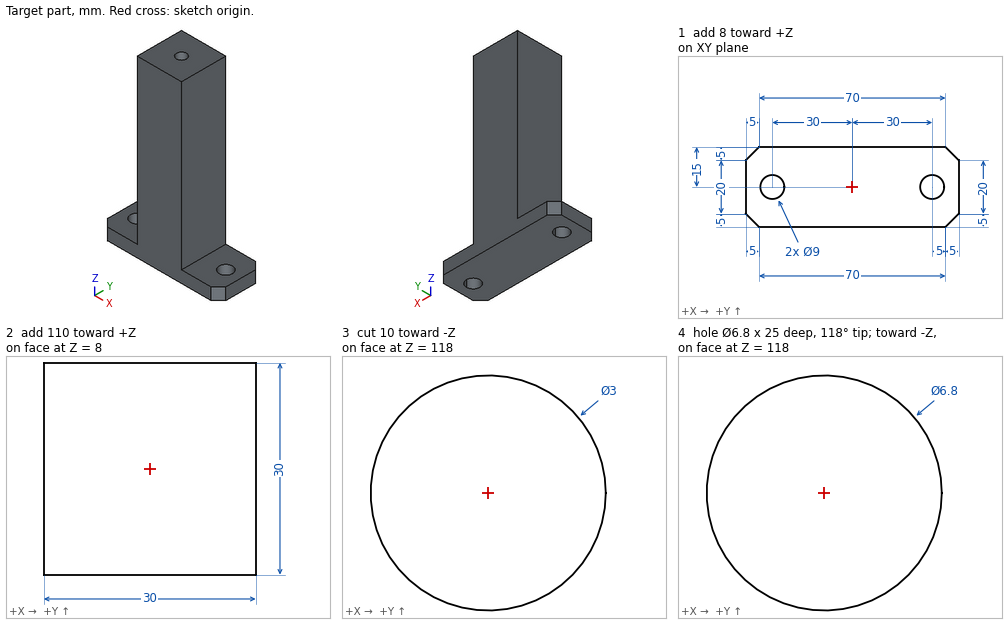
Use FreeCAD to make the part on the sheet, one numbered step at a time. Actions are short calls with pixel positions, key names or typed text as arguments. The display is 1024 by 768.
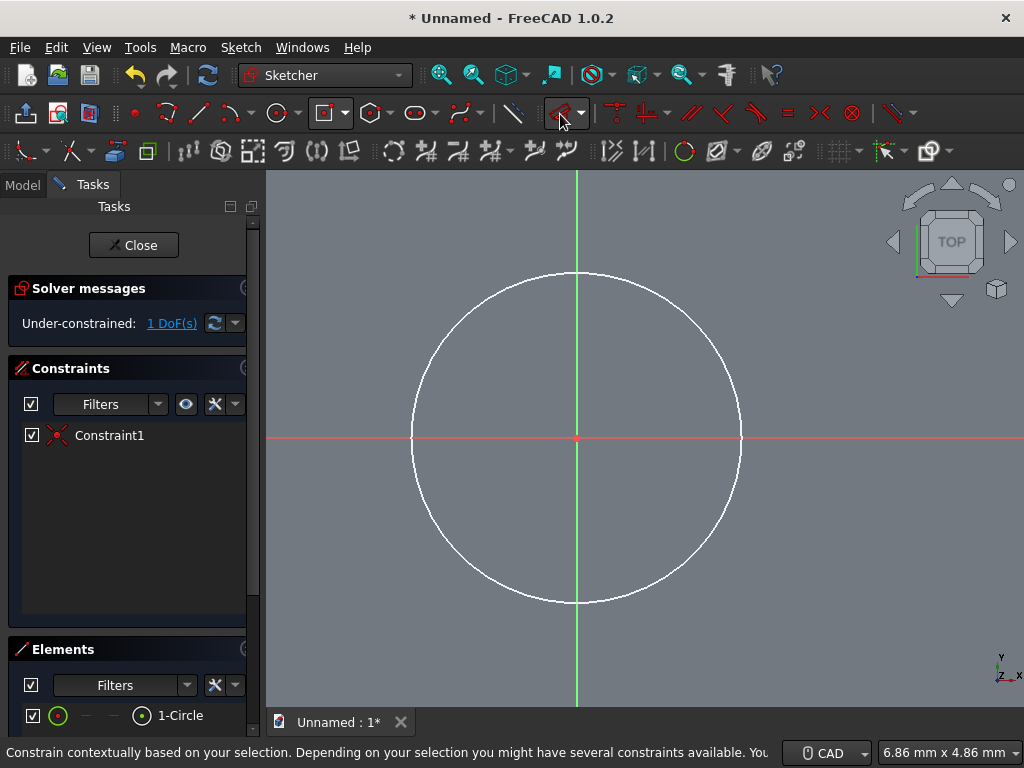
click(693, 321)
click(716, 298)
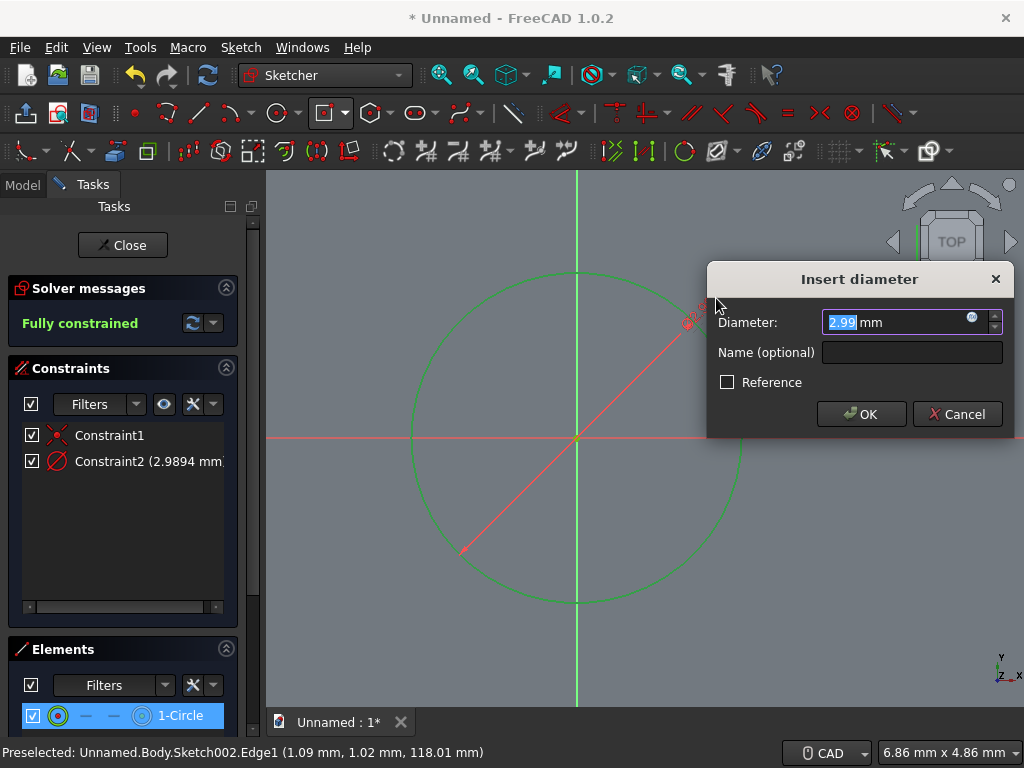
text(3)
key(Return)
key(Escape)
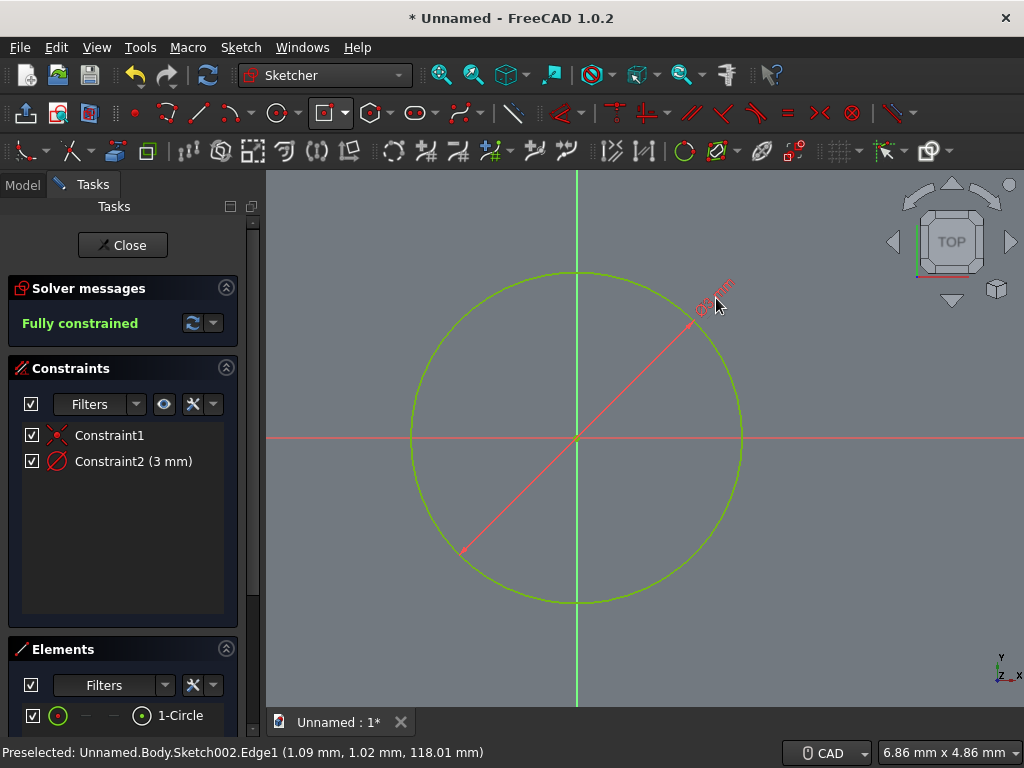
click(123, 245)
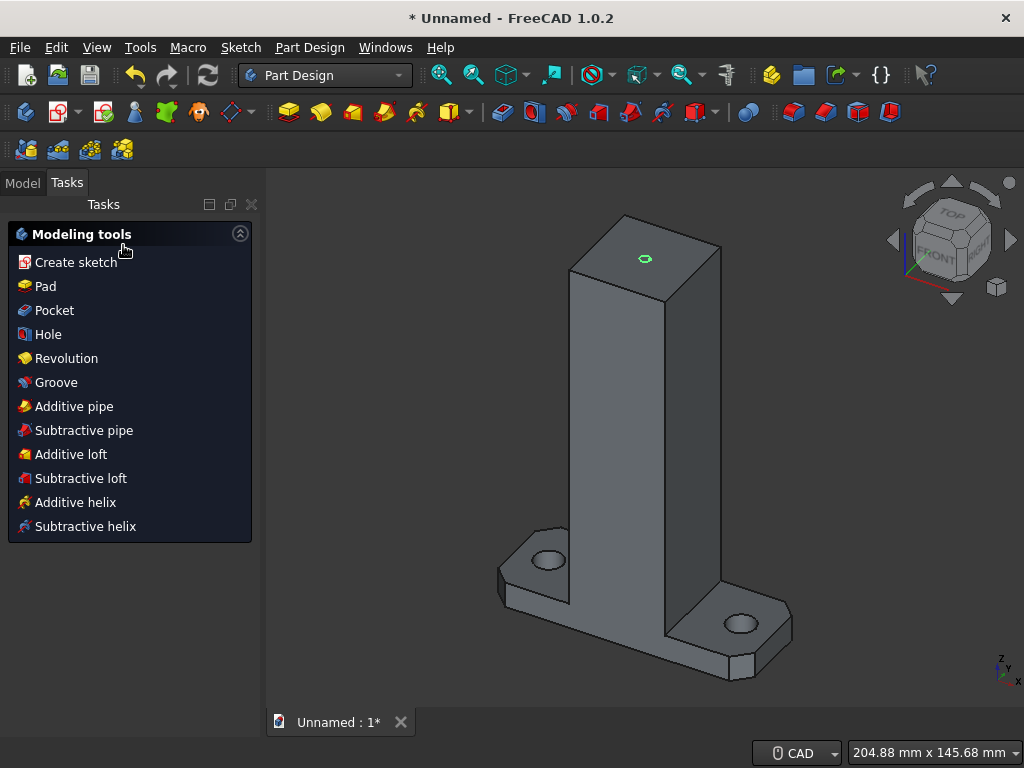
click(504, 112)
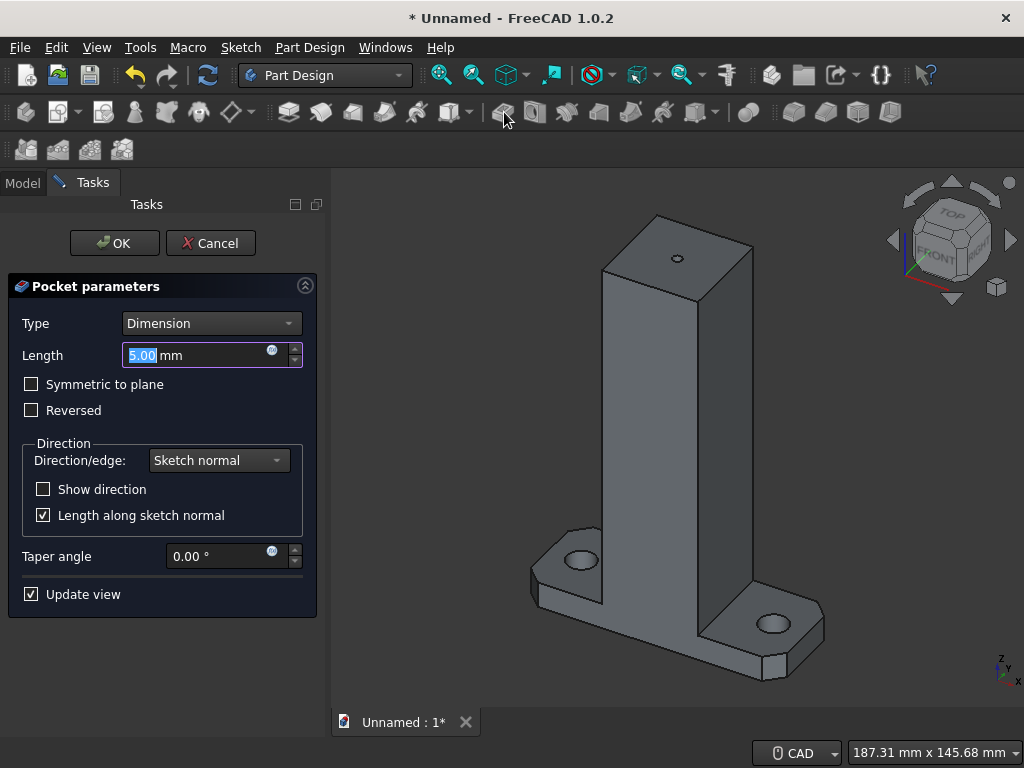
text(10)
key(Tab)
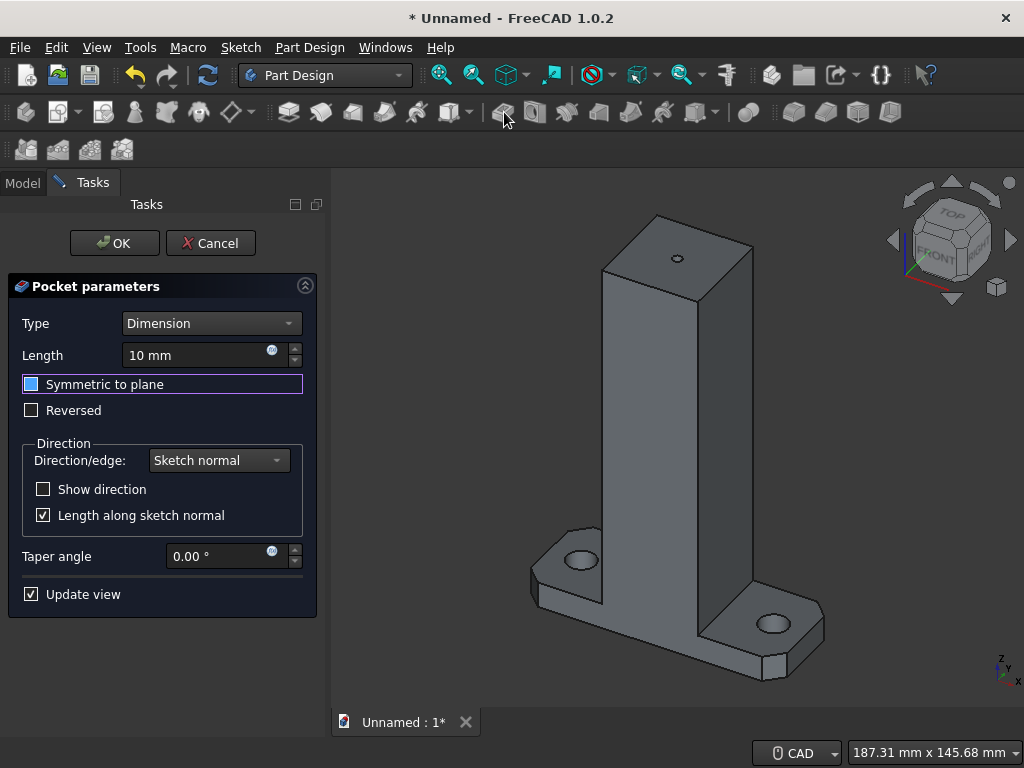
click(115, 243)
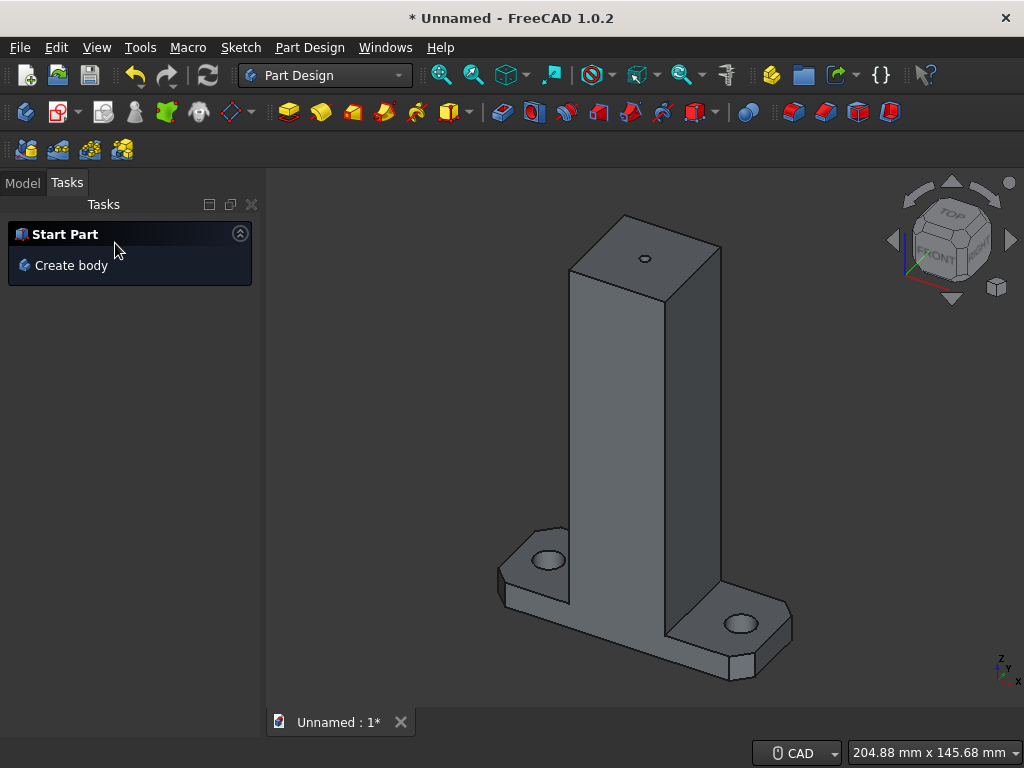
click(643, 278)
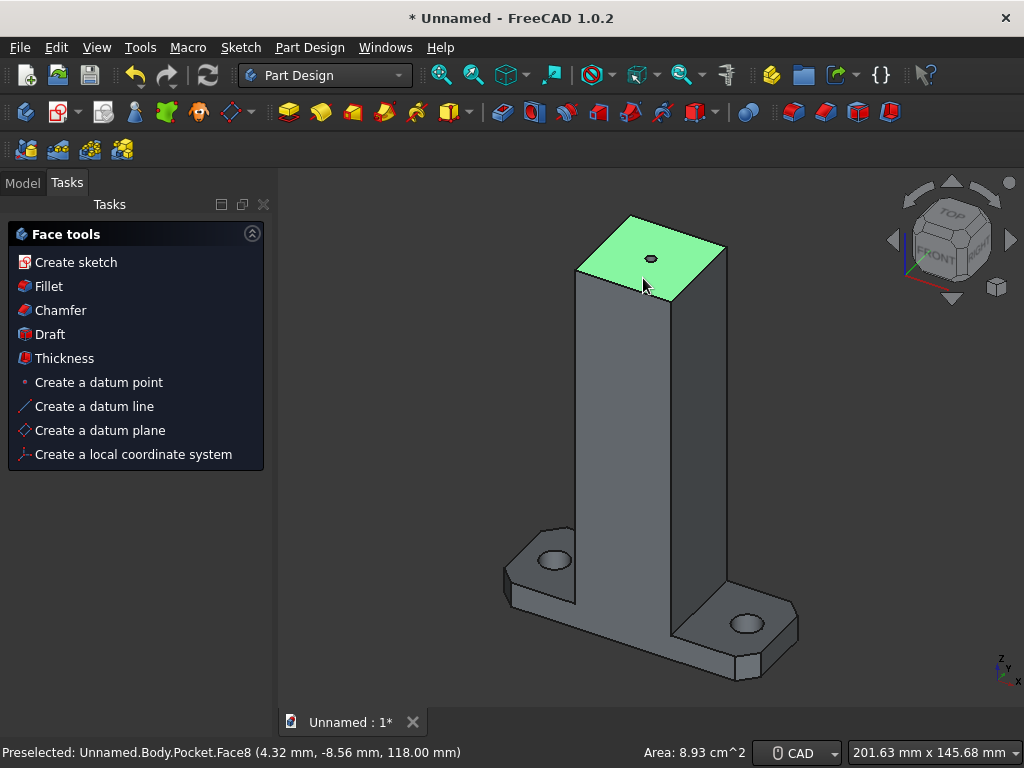
click(58, 112)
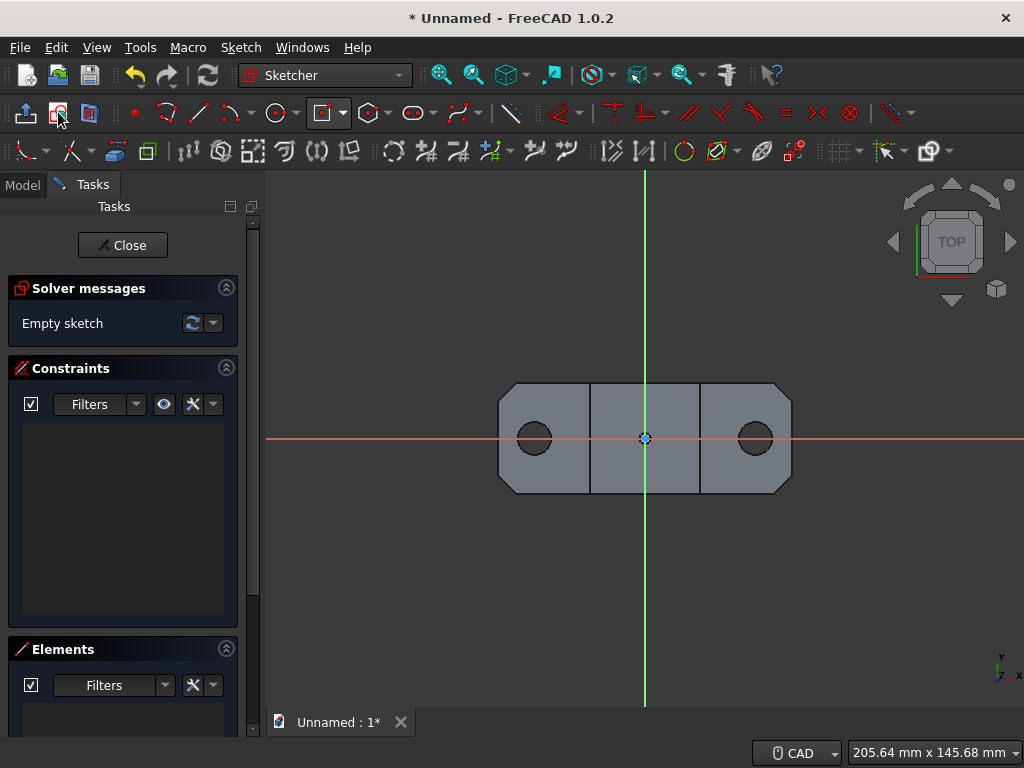
scroll(650, 438, up, 13)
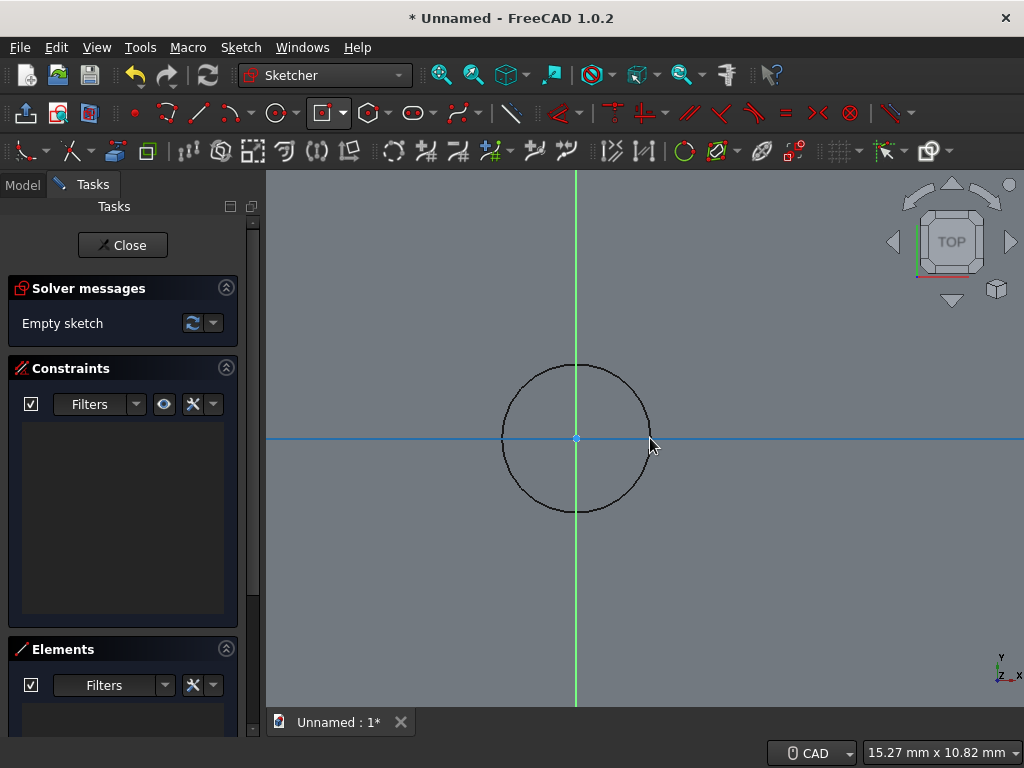
key(g)
key(c)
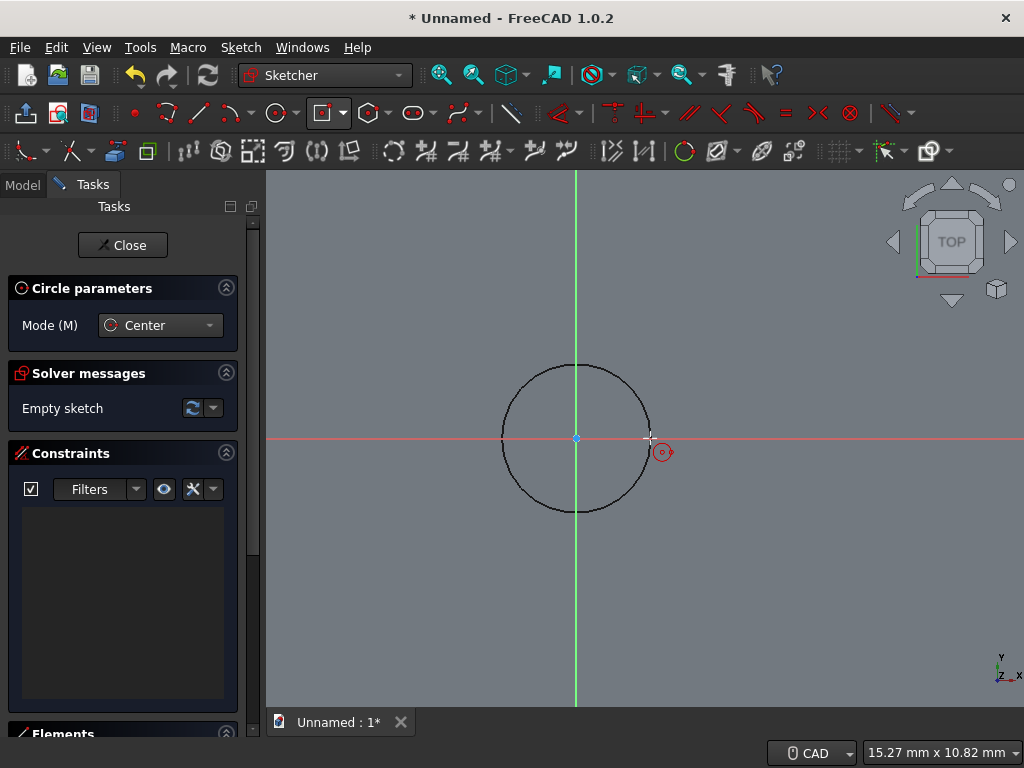
click(576, 438)
click(696, 319)
key(Escape)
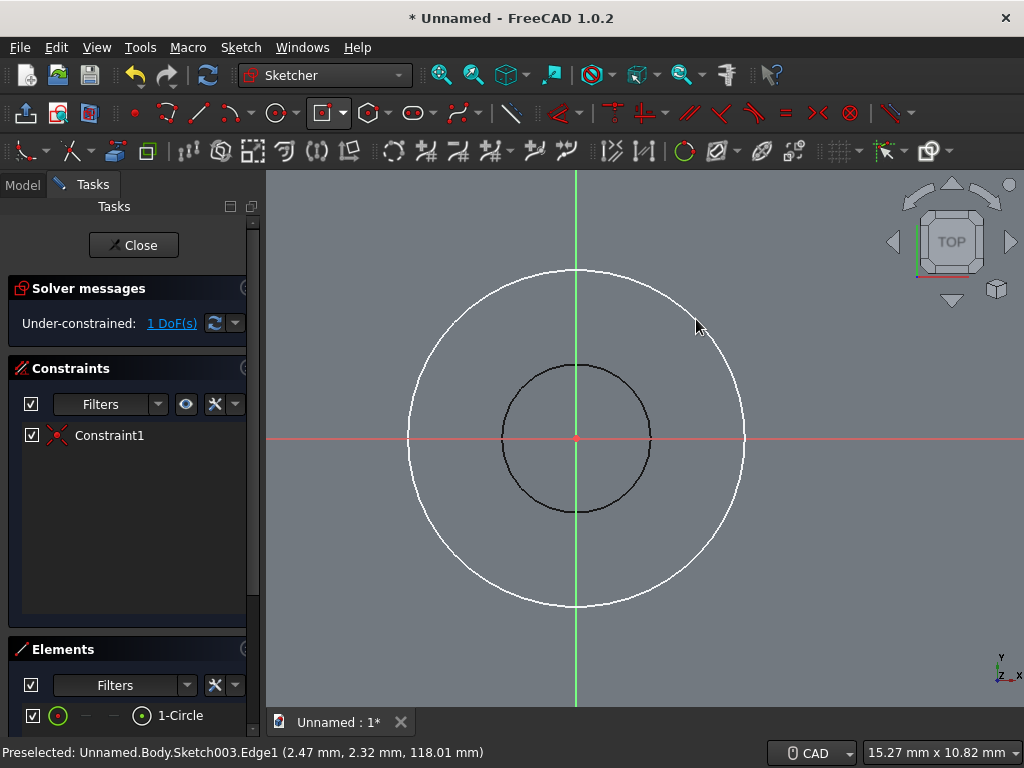
key(d)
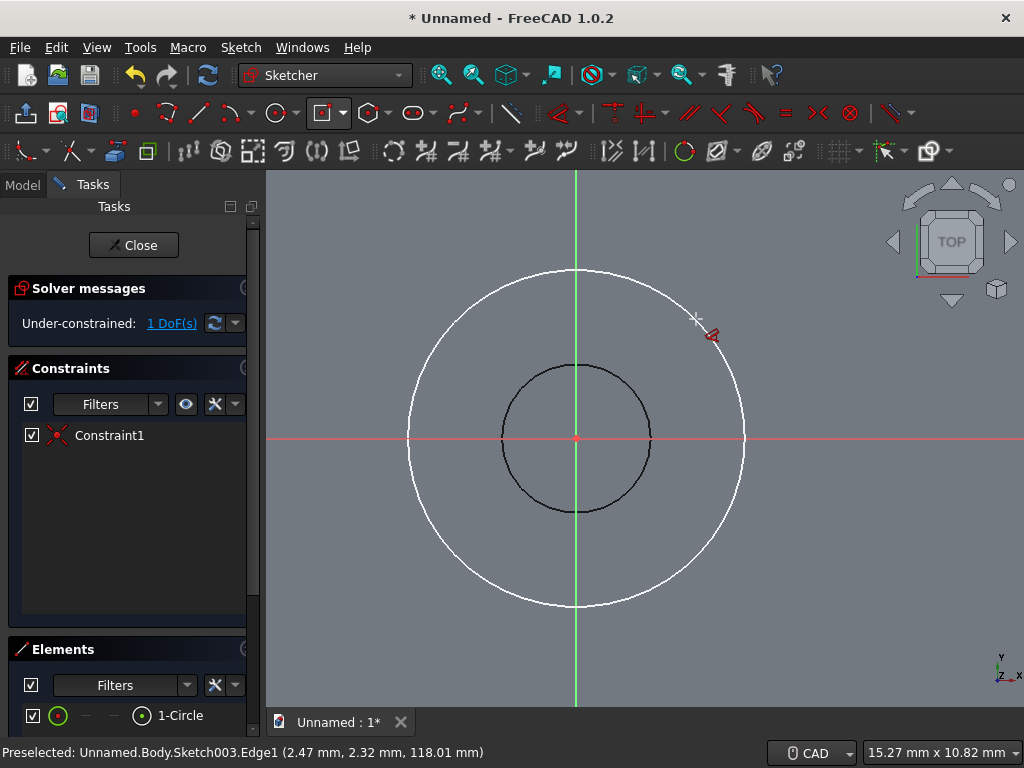
click(695, 319)
click(718, 296)